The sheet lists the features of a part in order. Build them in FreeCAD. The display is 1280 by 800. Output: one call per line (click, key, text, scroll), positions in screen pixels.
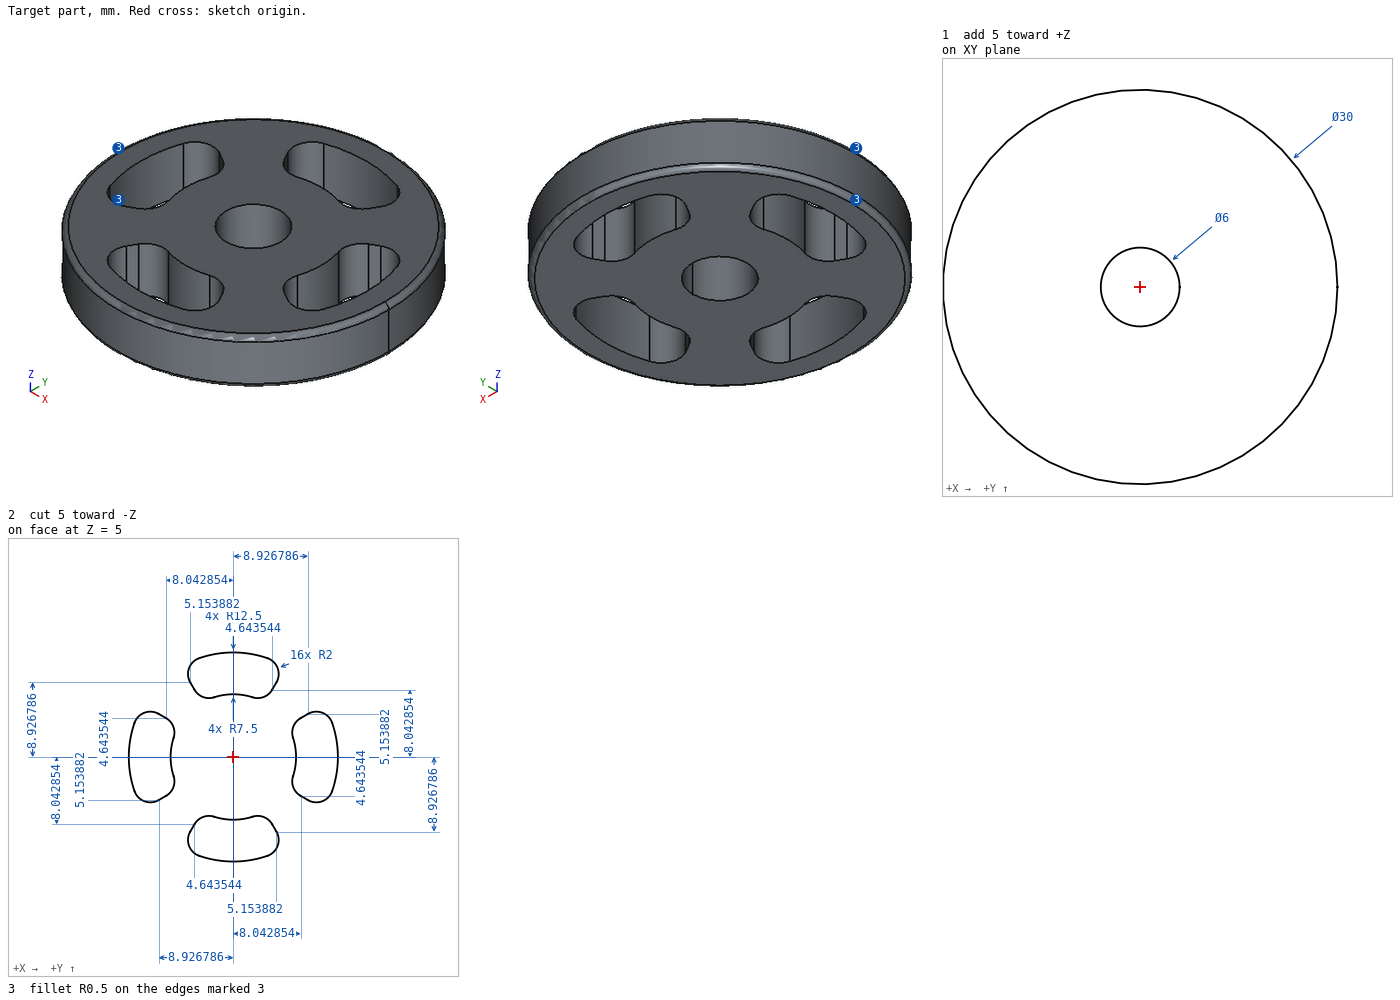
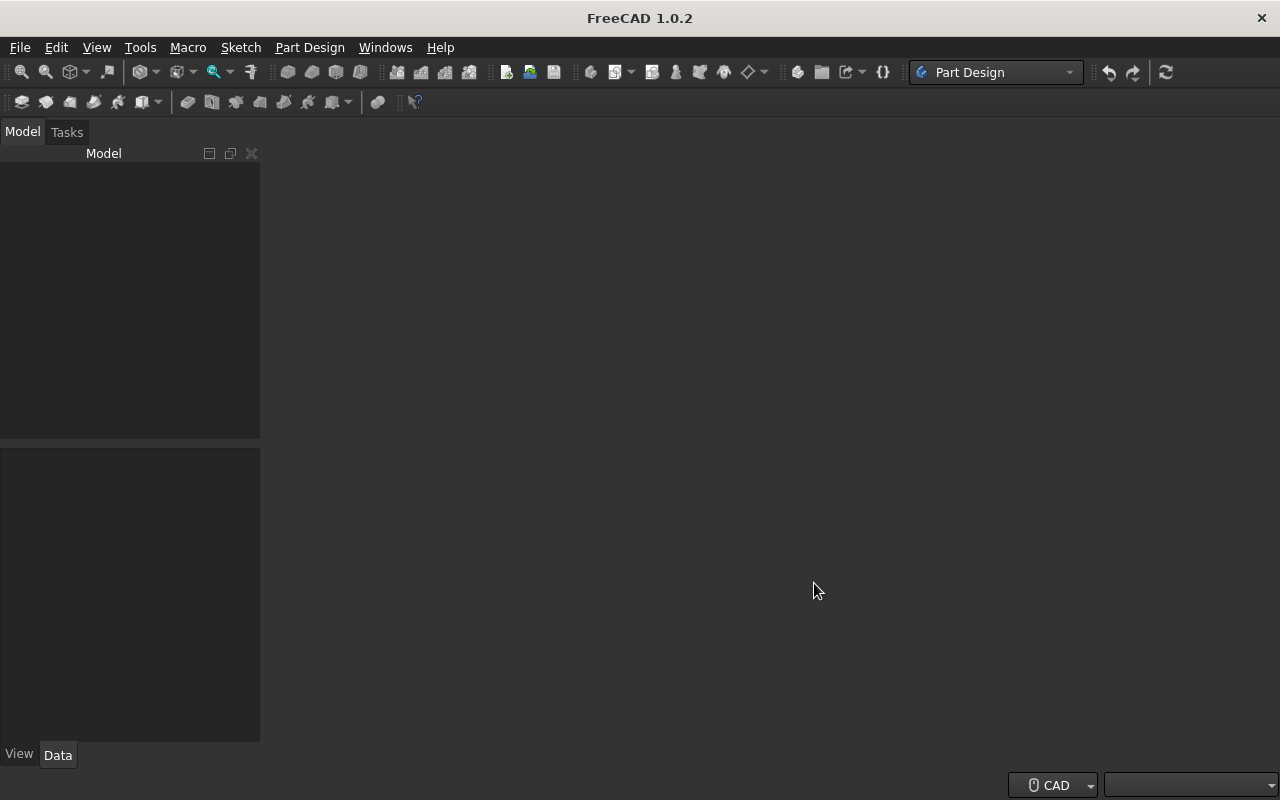
click(506, 72)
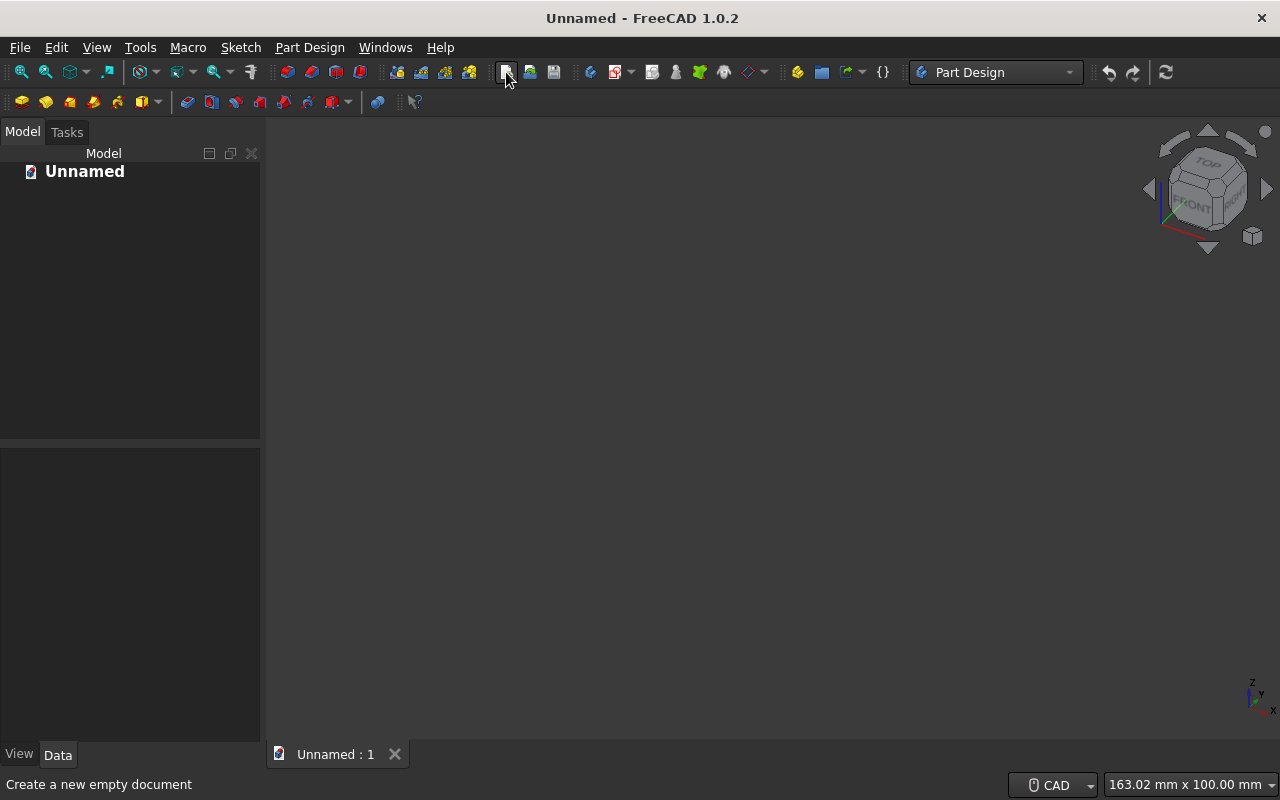
click(616, 72)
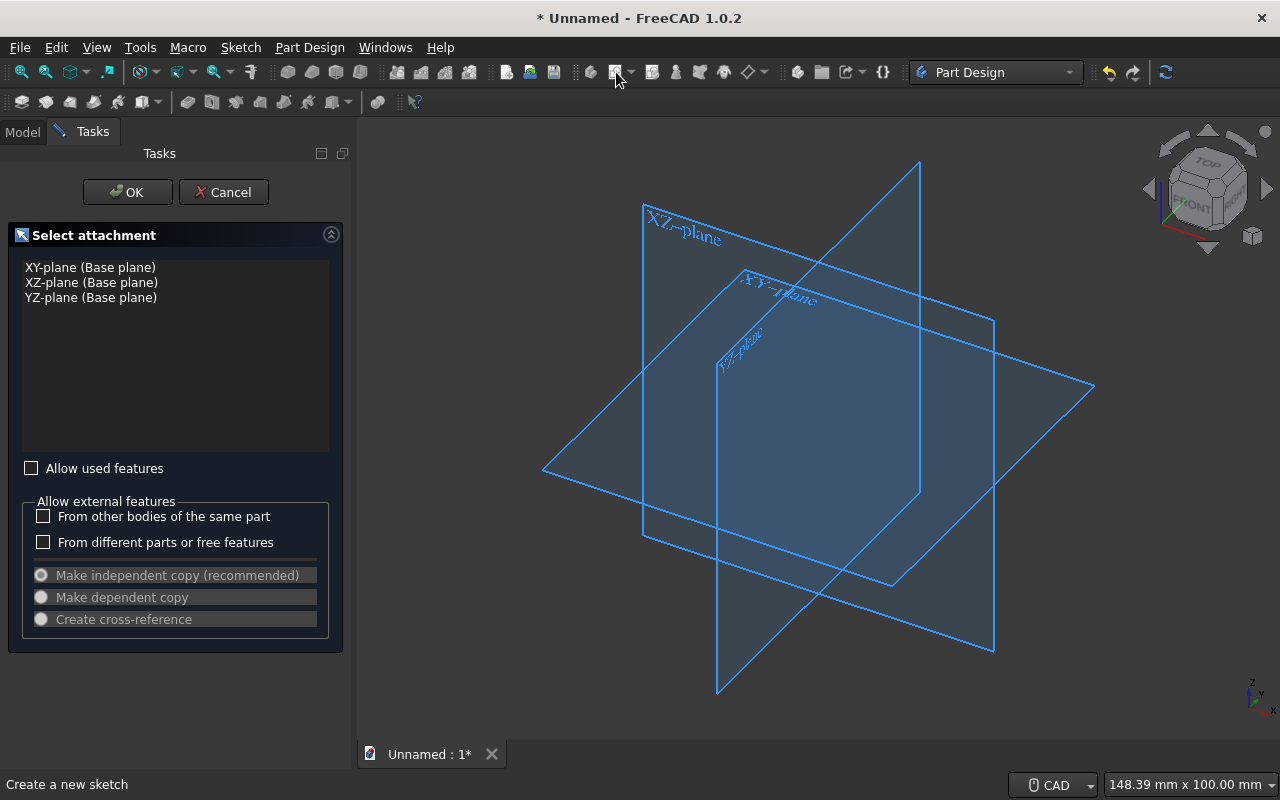
click(82, 268)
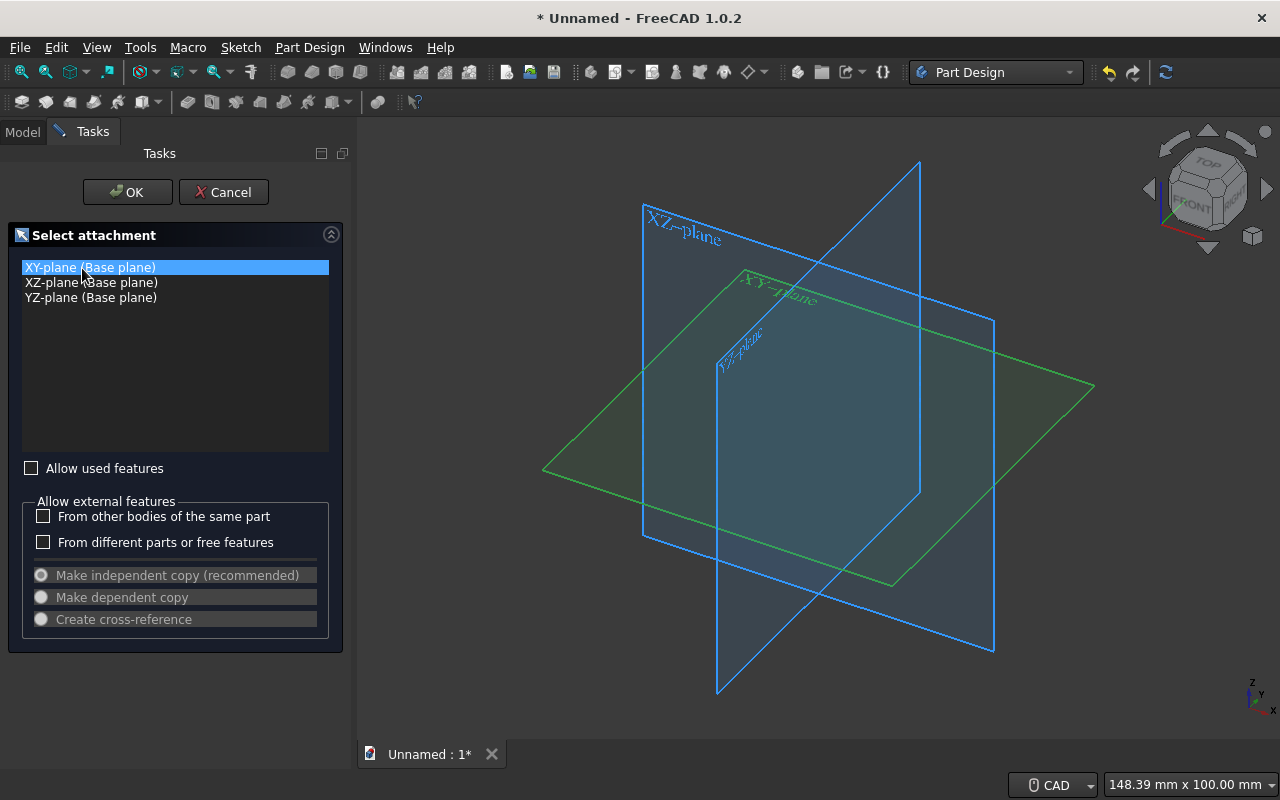
click(128, 192)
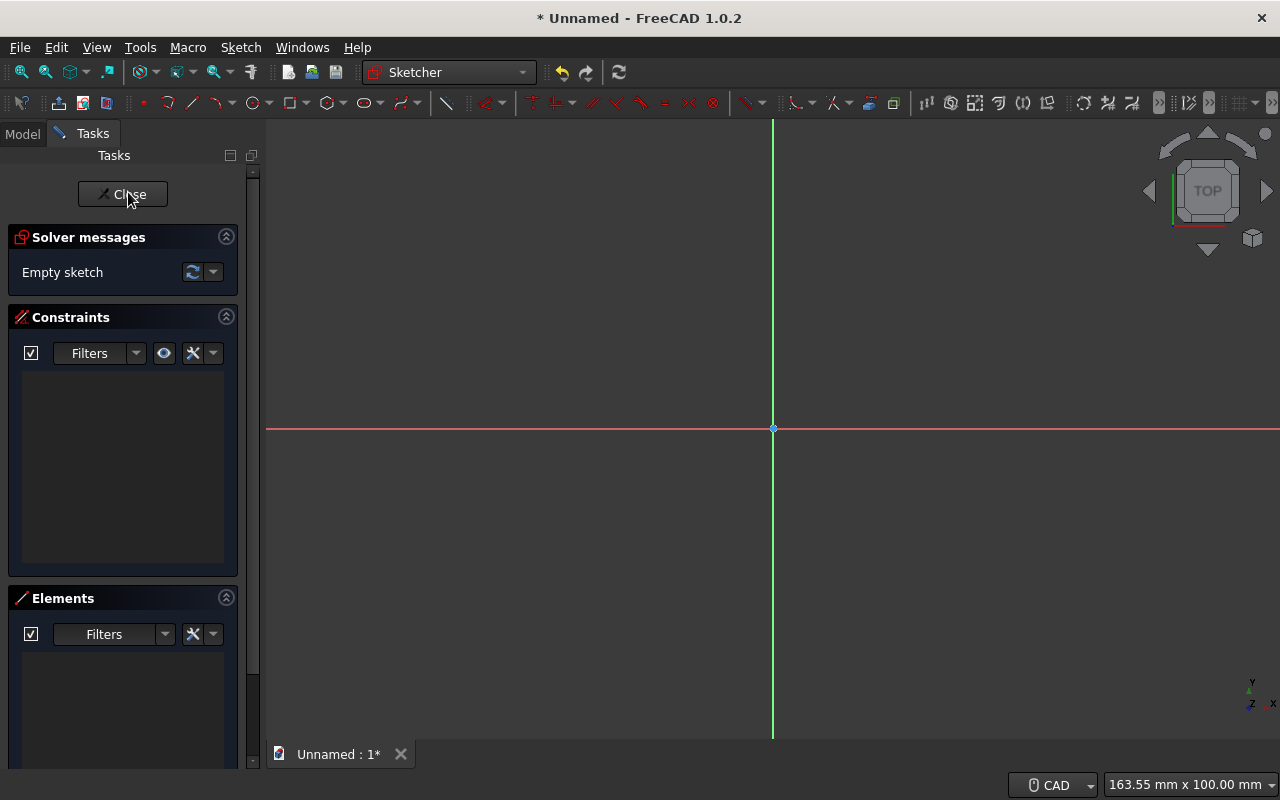
scroll(829, 429, up, 4)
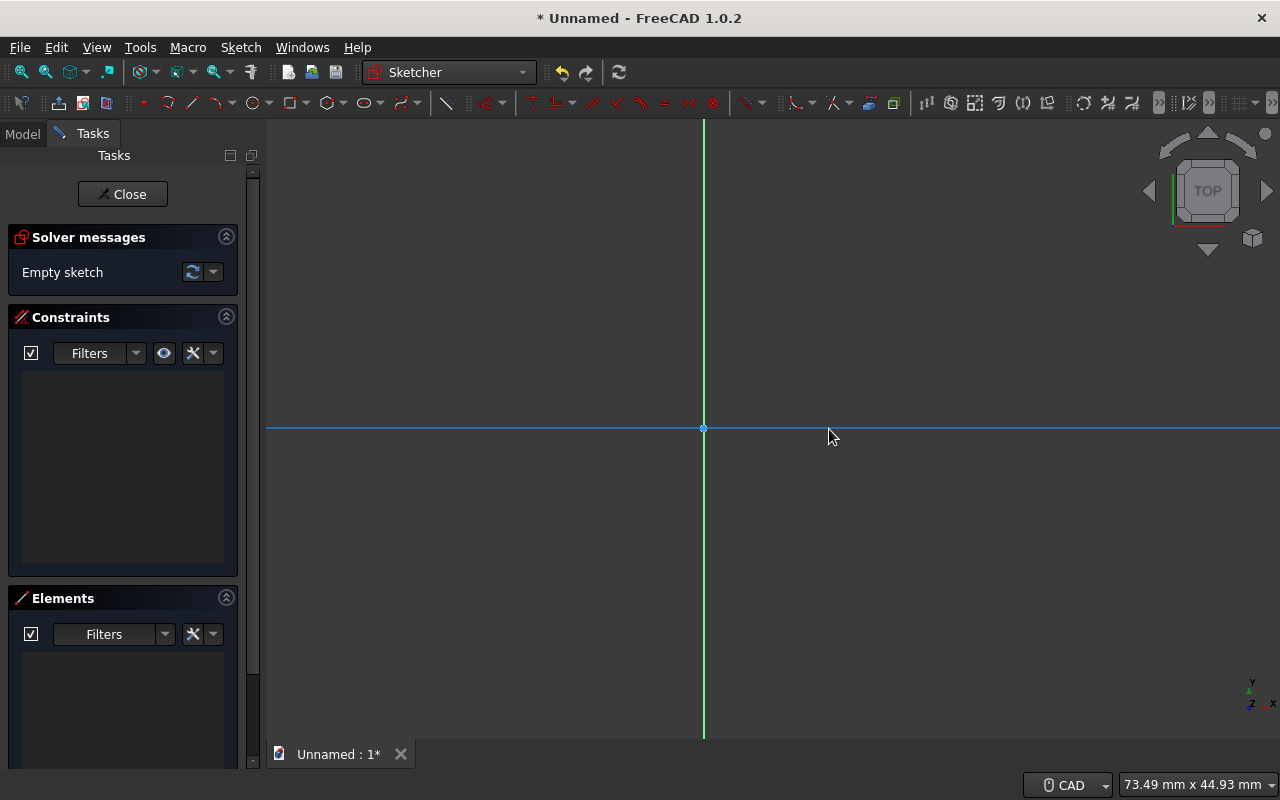
click(254, 104)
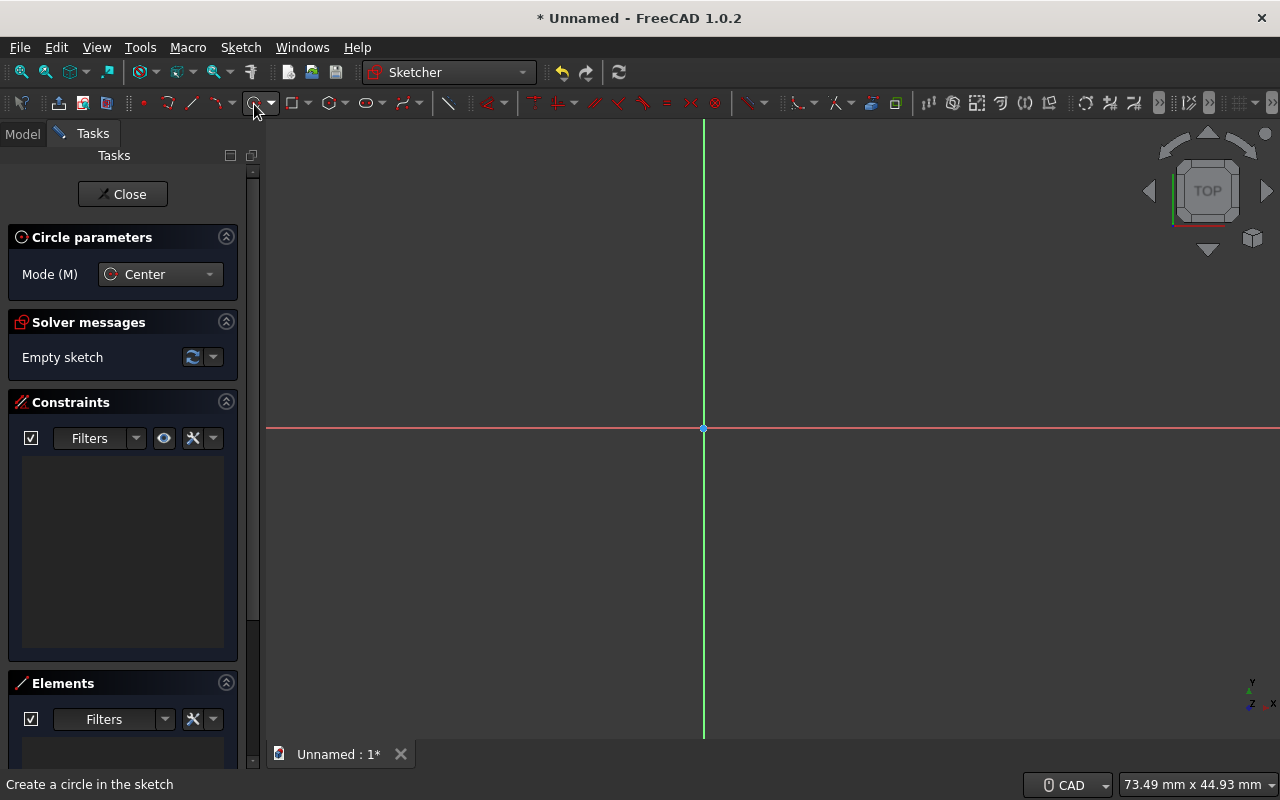
click(704, 428)
click(850, 282)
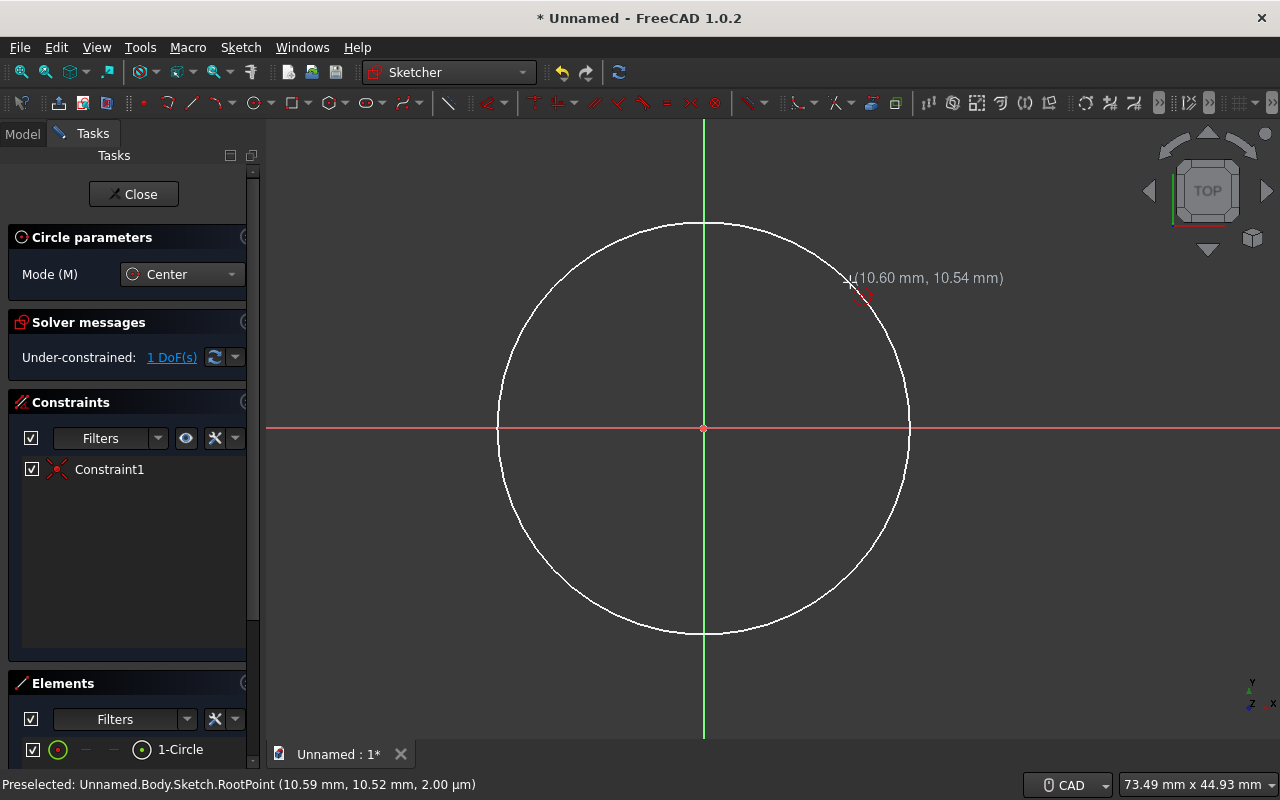
click(704, 428)
click(733, 399)
key(Escape)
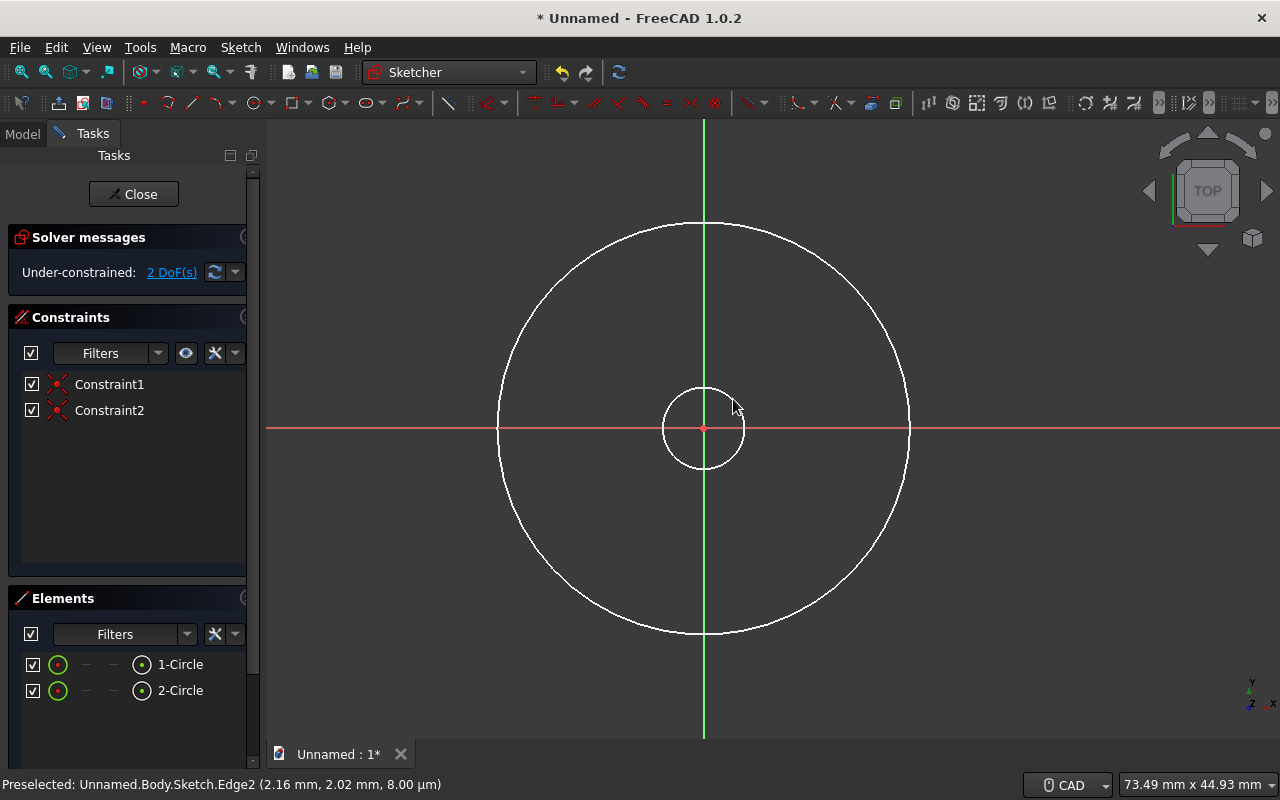
click(849, 282)